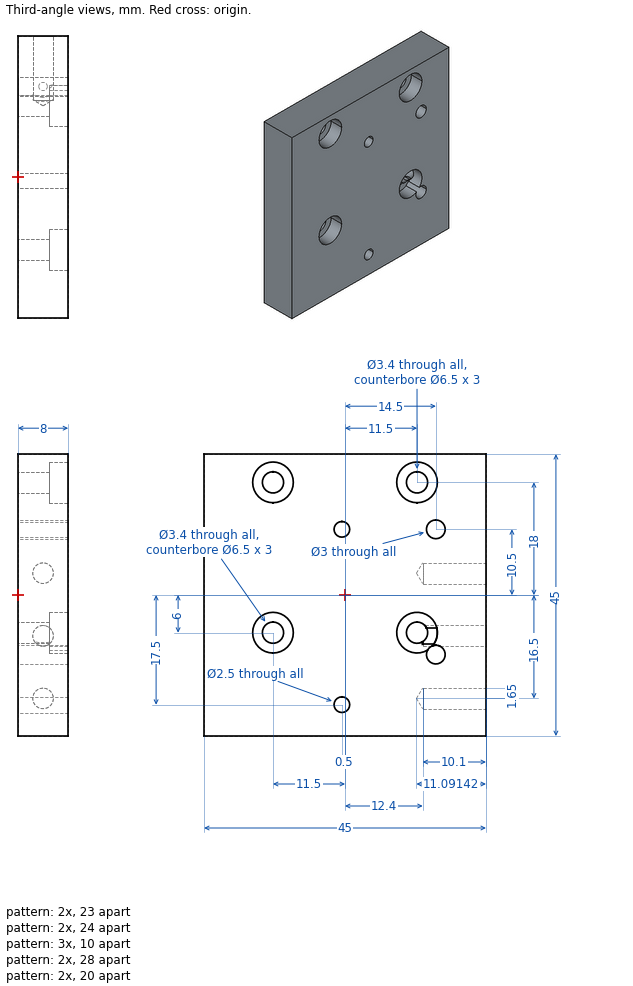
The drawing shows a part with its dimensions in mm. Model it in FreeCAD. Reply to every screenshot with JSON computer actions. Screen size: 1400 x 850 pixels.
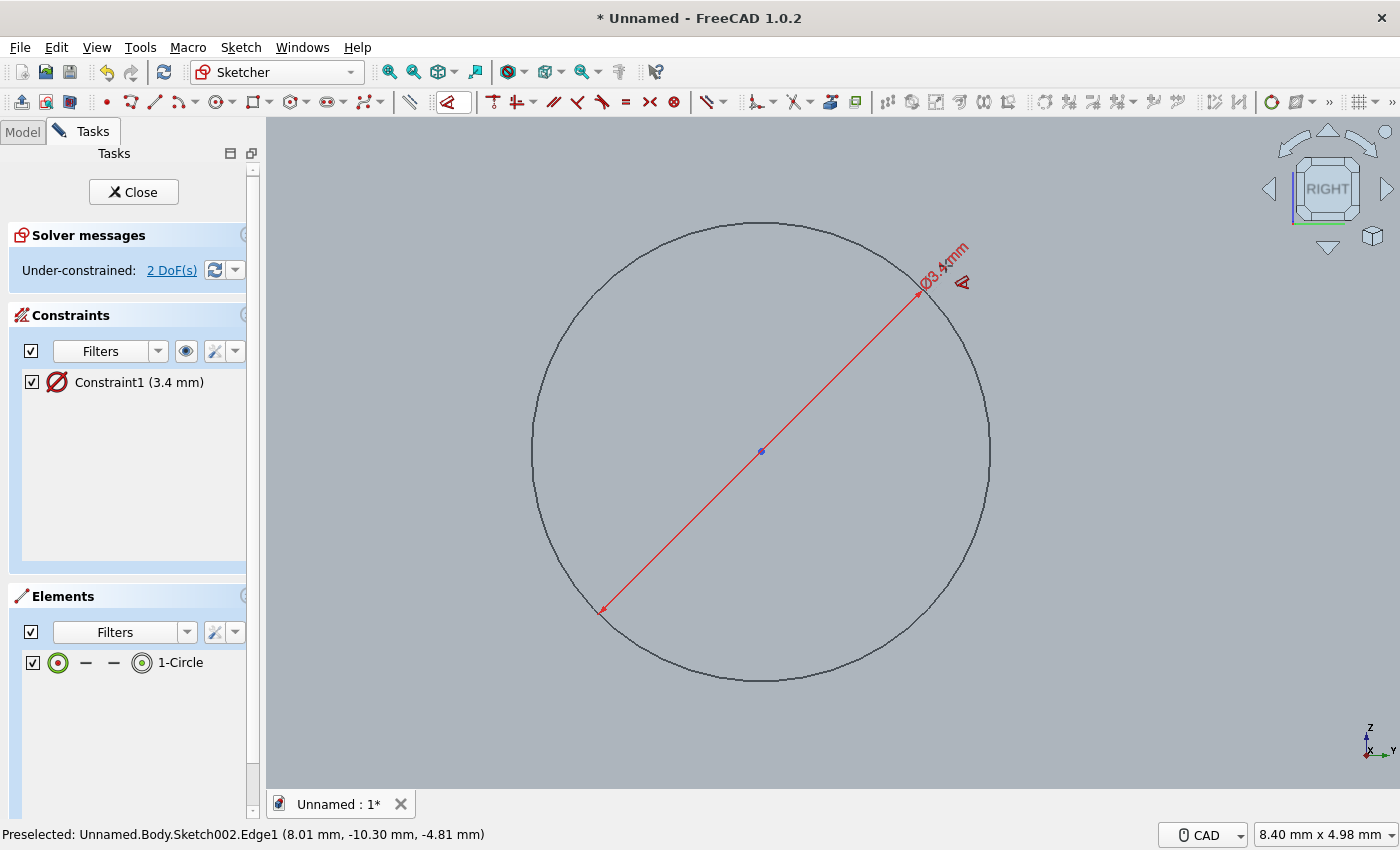
{"action": "left_click", "coordinate": [761, 452]}
{"action": "left_click", "coordinate": [727, 299]}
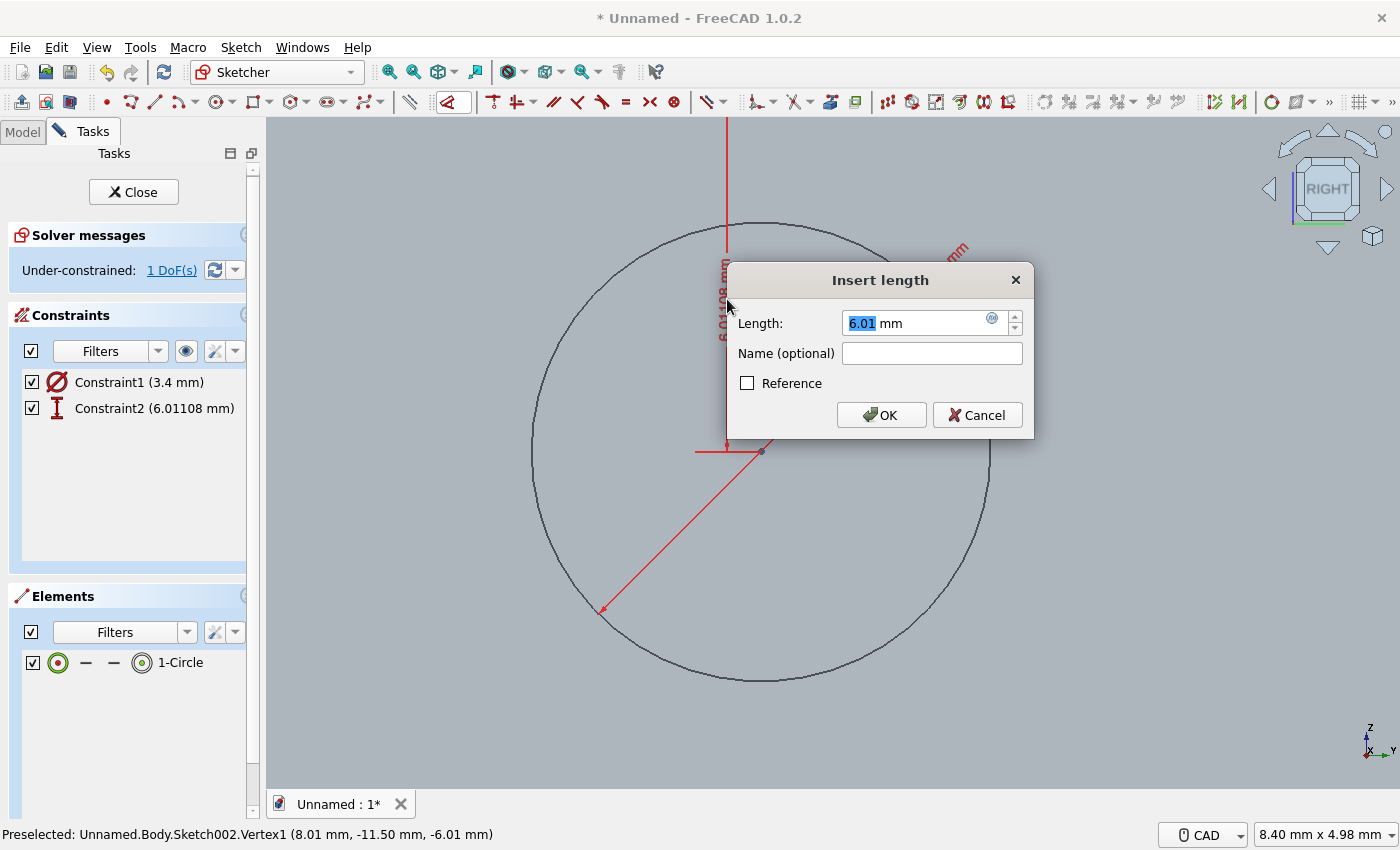
{"action": "type", "text": "6"}
{"action": "key", "text": "Return"}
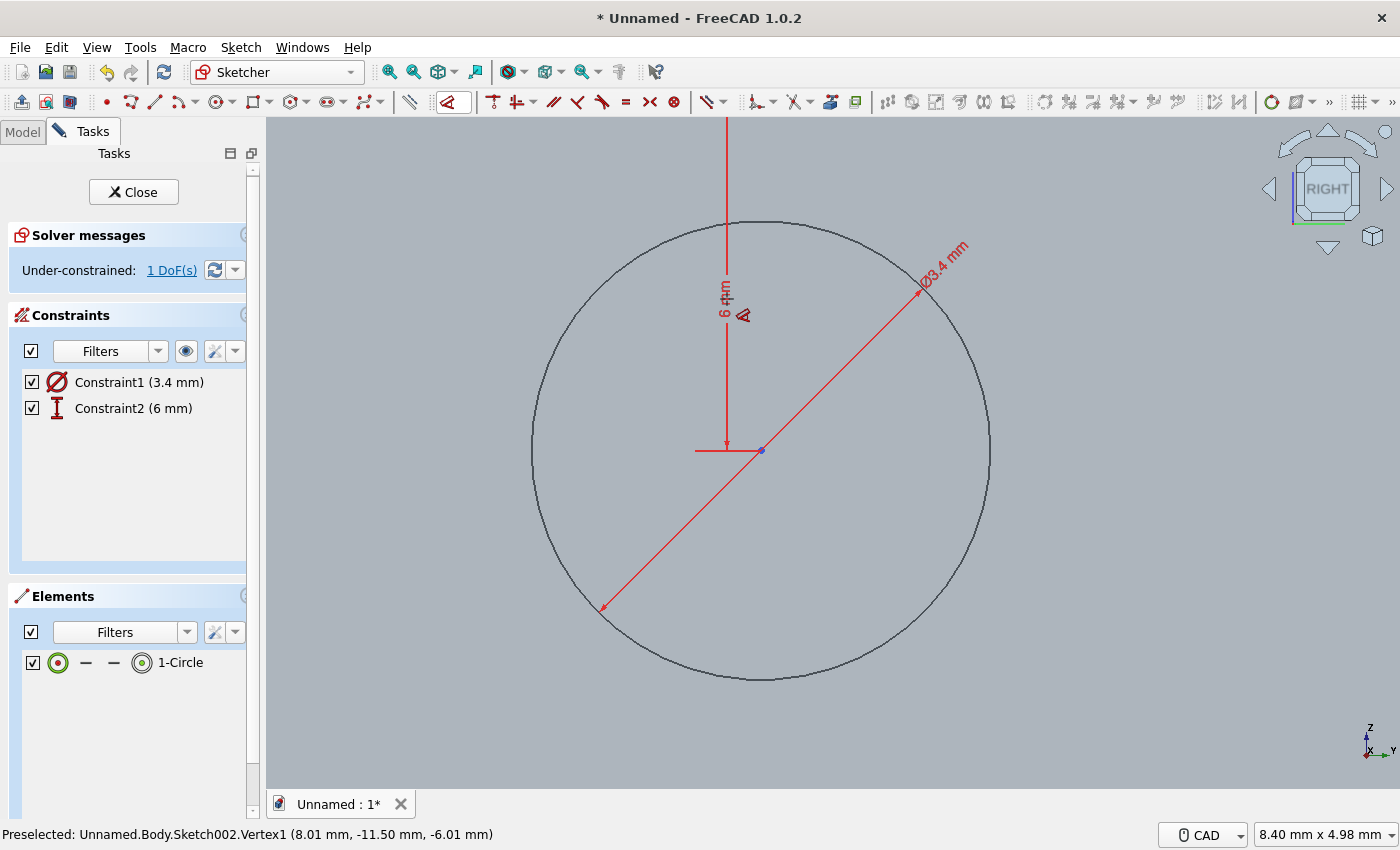
{"action": "left_click", "coordinate": [761, 451]}
{"action": "left_click", "coordinate": [889, 485]}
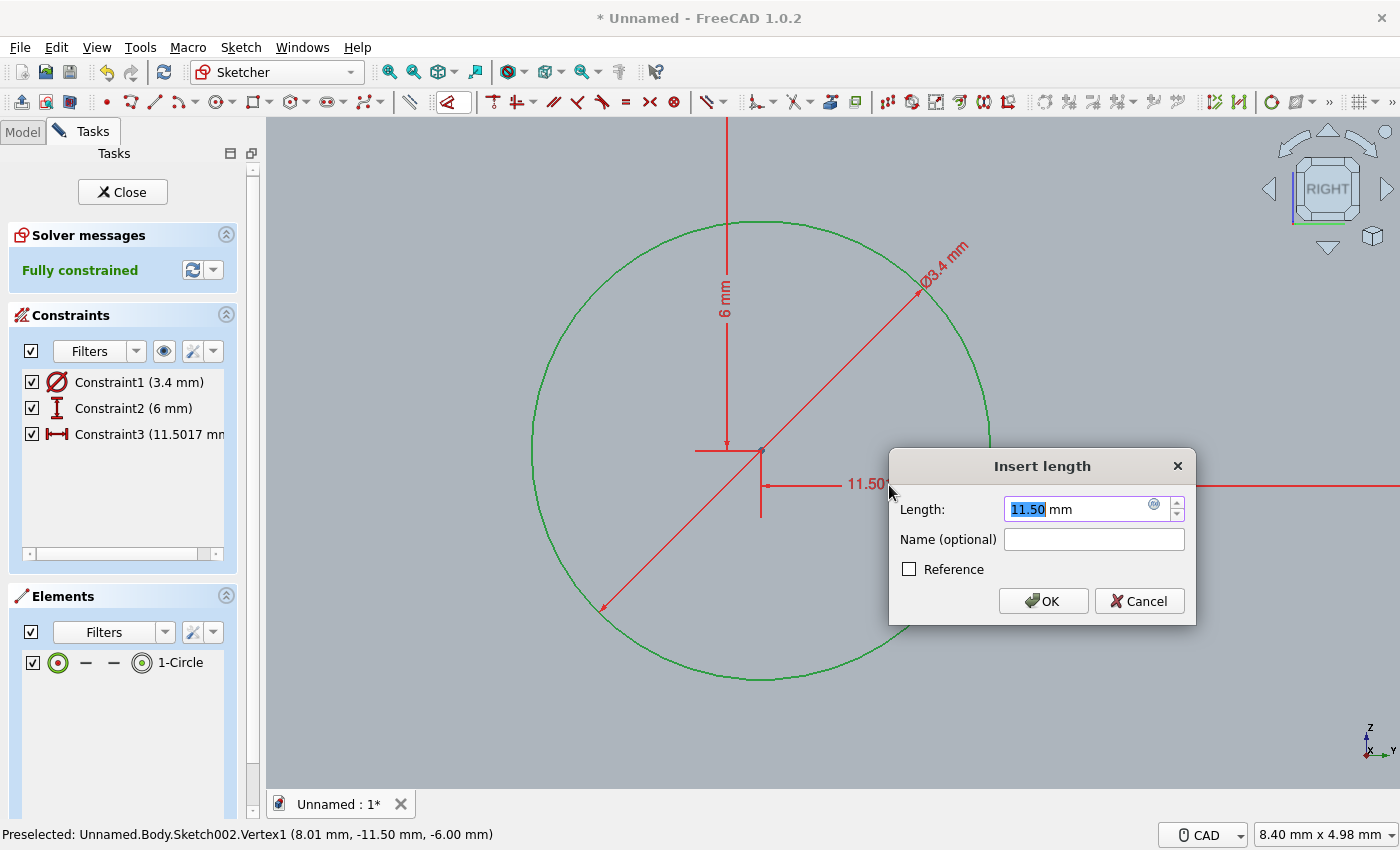
{"action": "type", "text": "11.5"}
{"action": "key", "text": "Return"}
{"action": "key", "text": "Escape"}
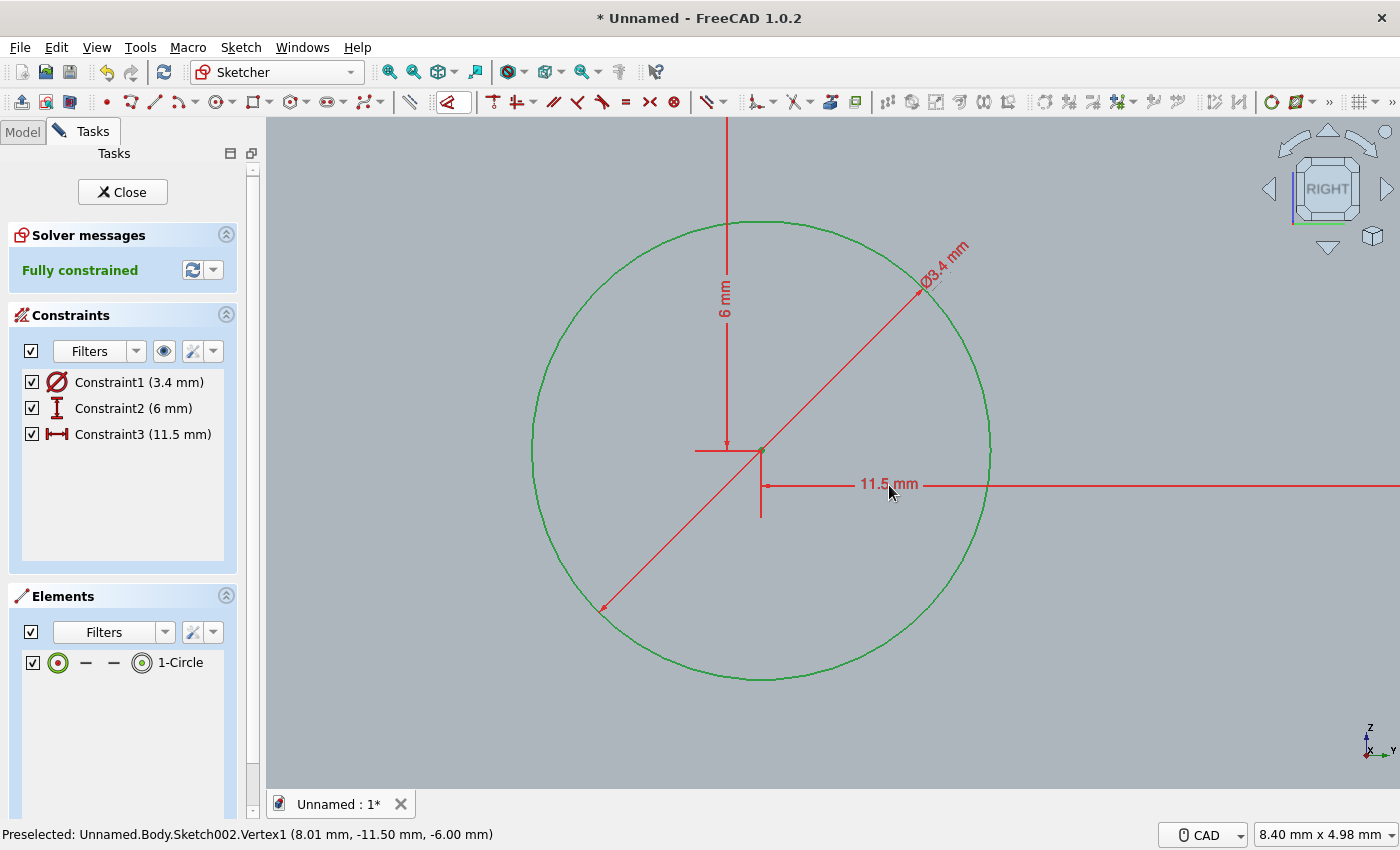
{"action": "left_click", "coordinate": [123, 192]}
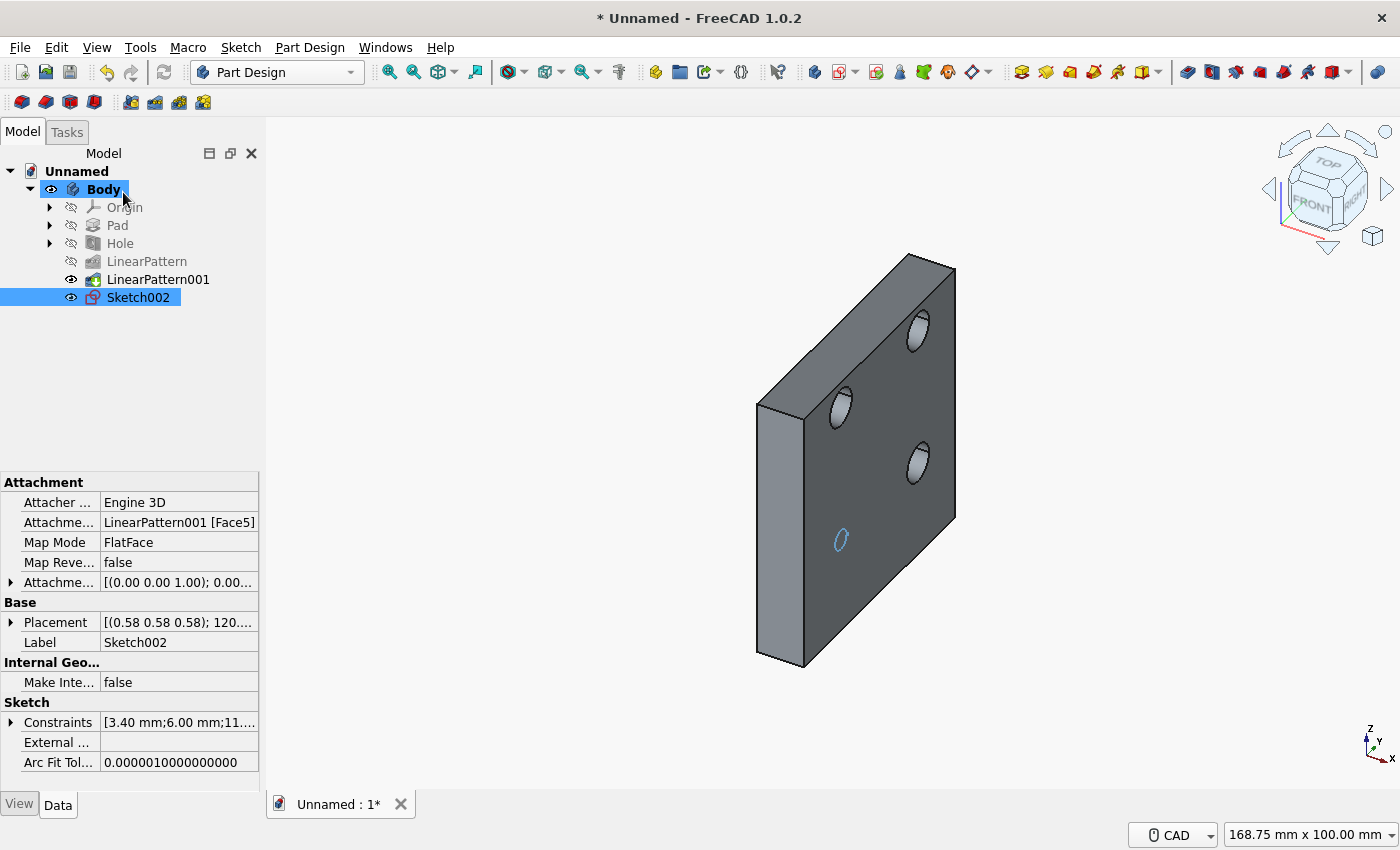
{"action": "left_click", "coordinate": [1212, 72]}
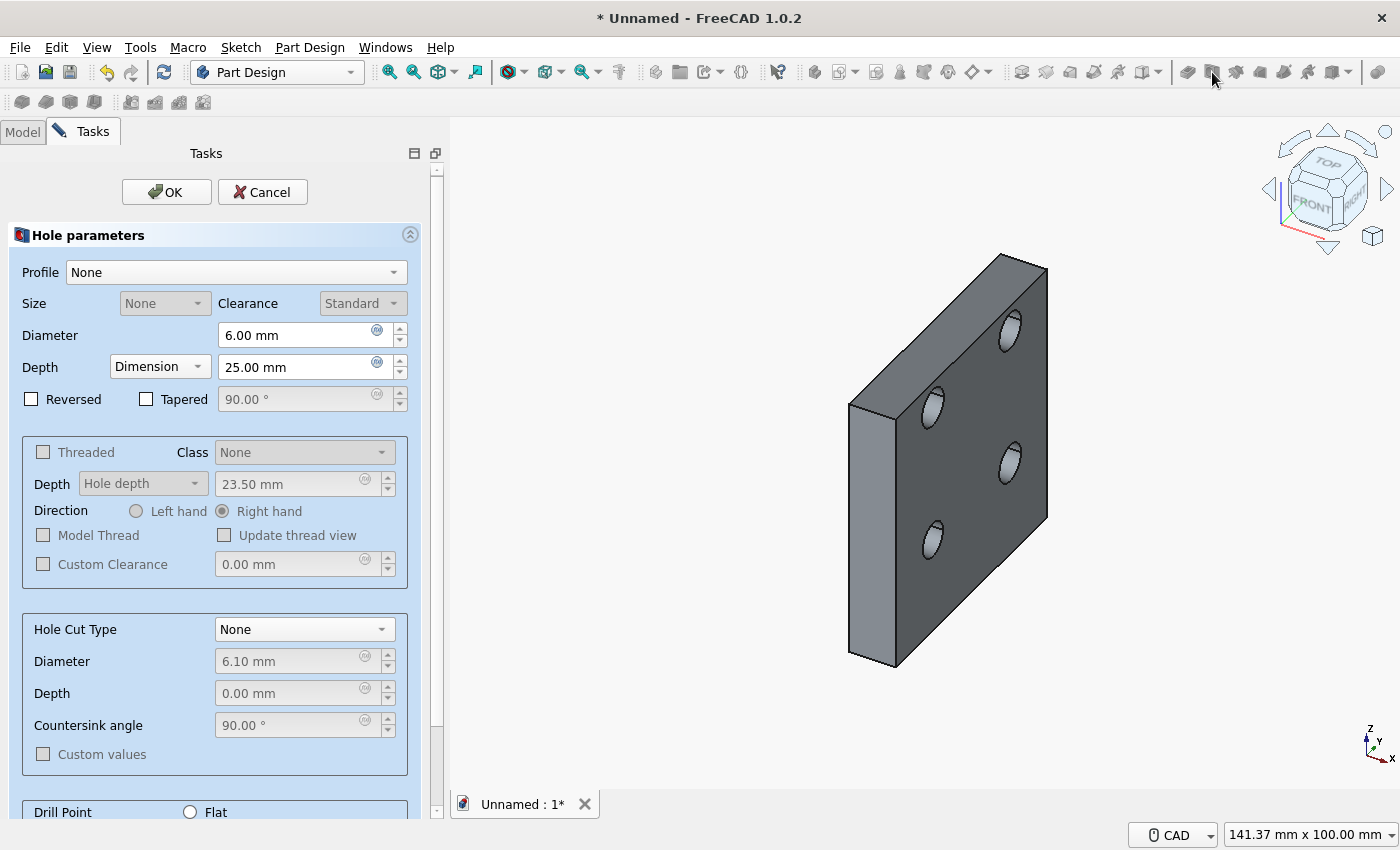
{"action": "triple_click", "coordinate": [305, 335]}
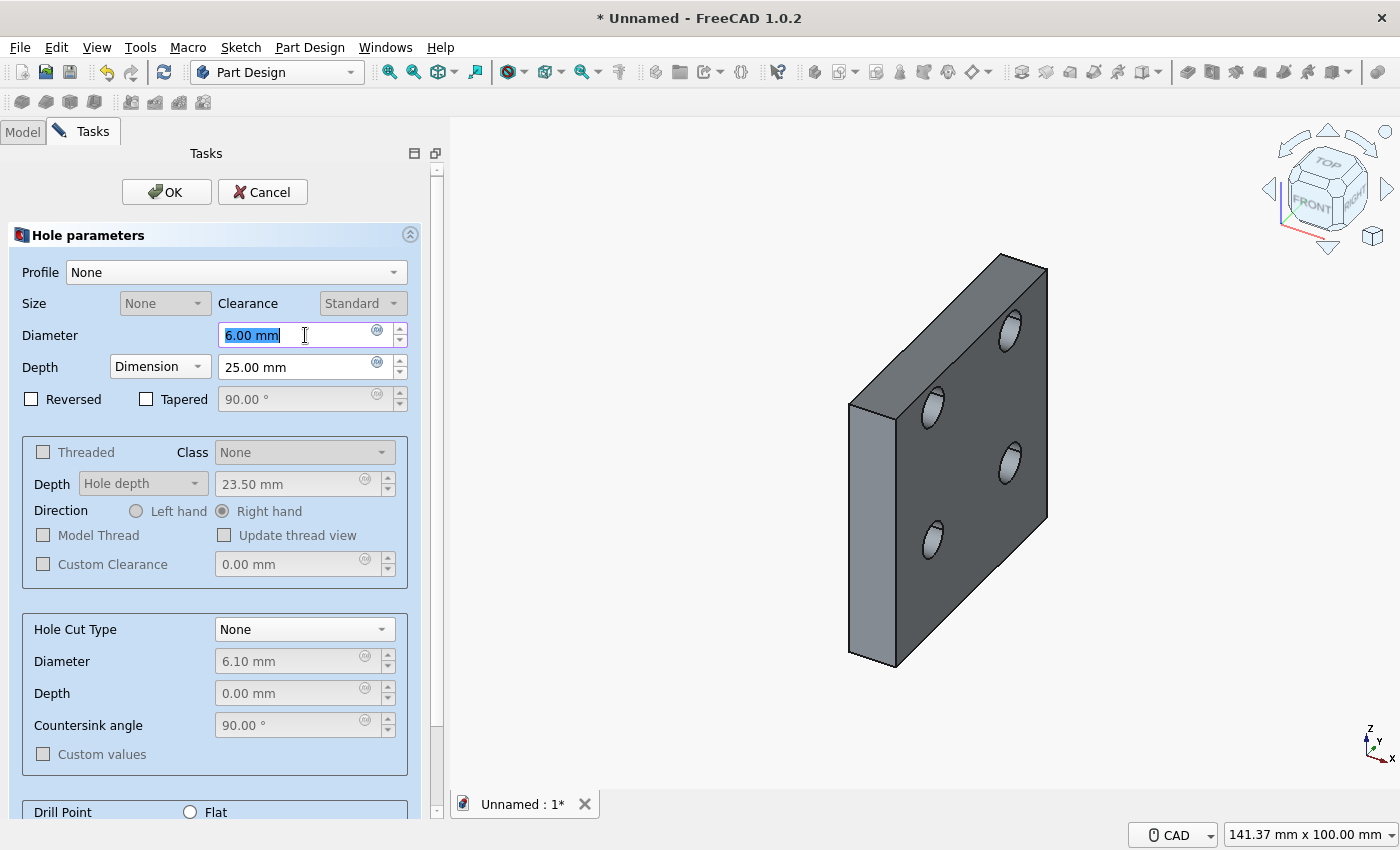
{"action": "type", "text": "3.4"}
{"action": "key", "text": "Tab"}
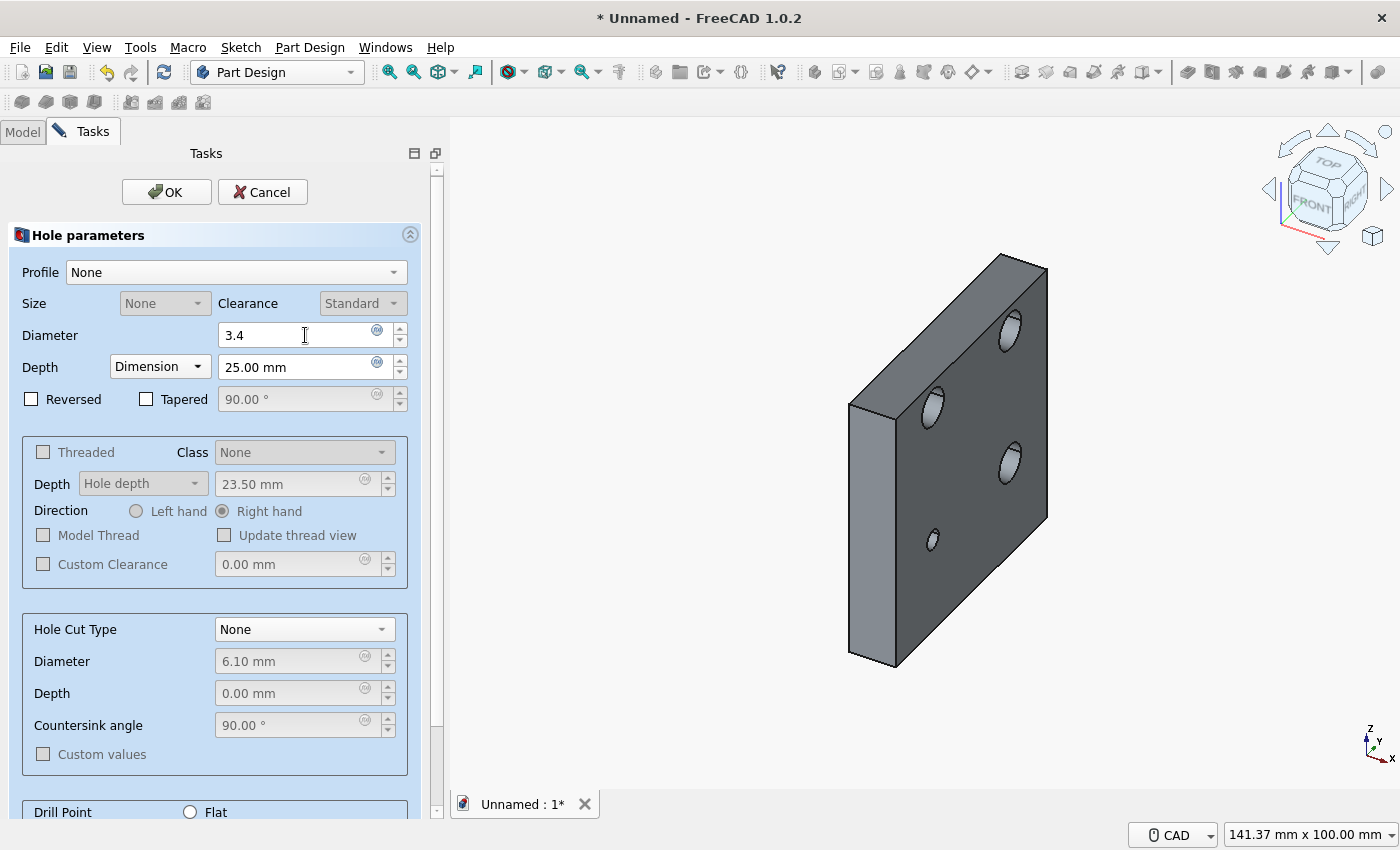
{"action": "left_click", "coordinate": [161, 366]}